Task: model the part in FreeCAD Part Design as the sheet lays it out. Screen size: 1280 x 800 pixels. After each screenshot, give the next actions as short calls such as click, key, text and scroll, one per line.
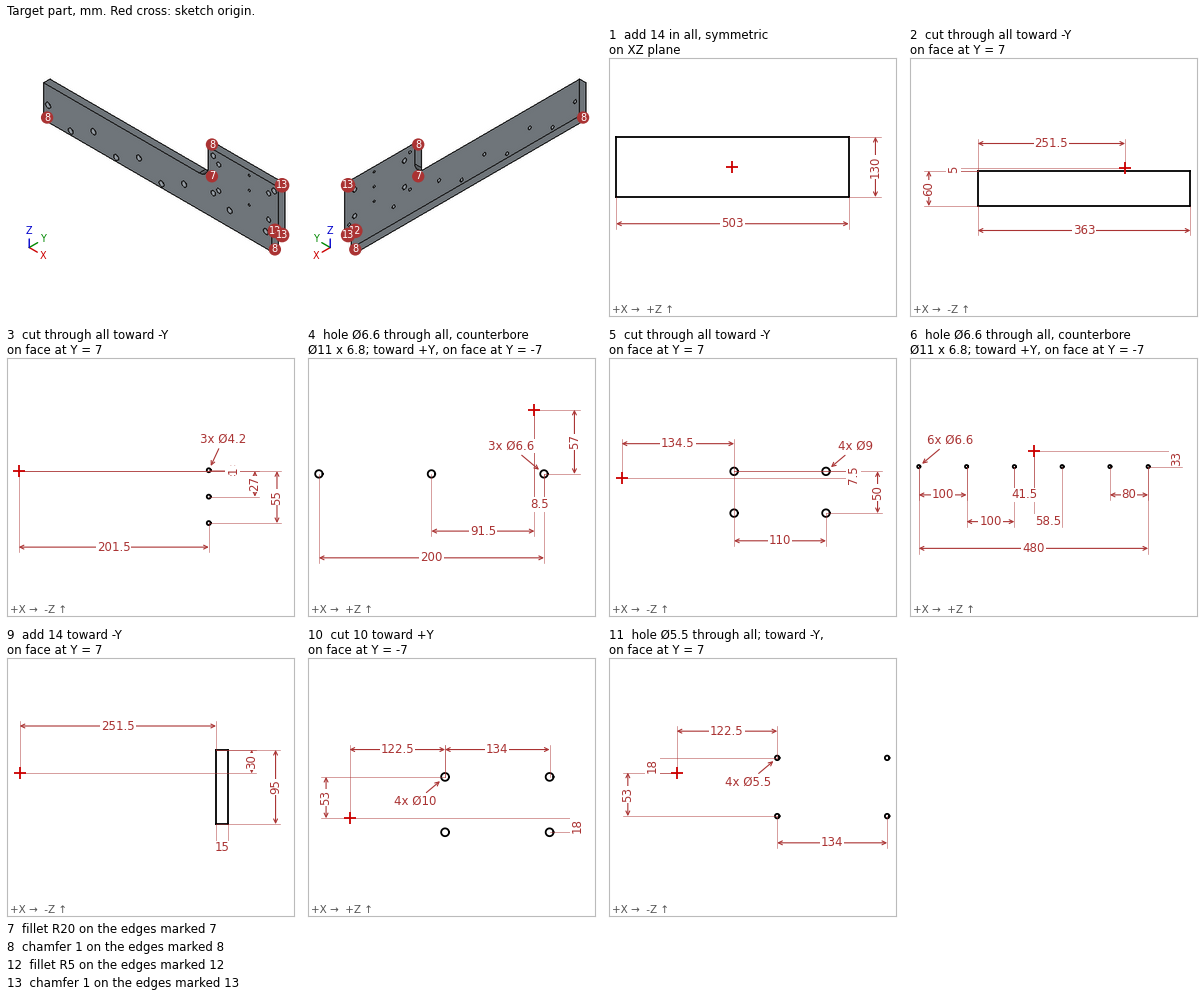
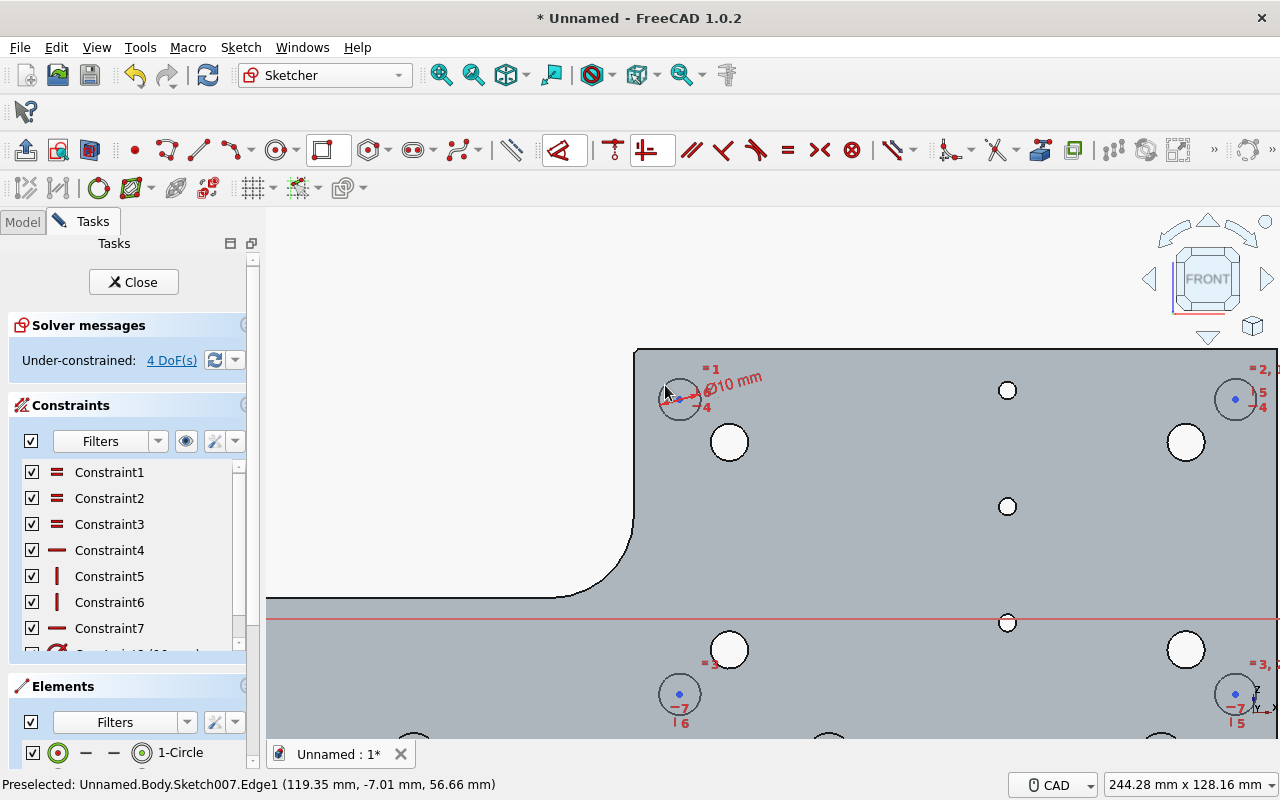
click(680, 400)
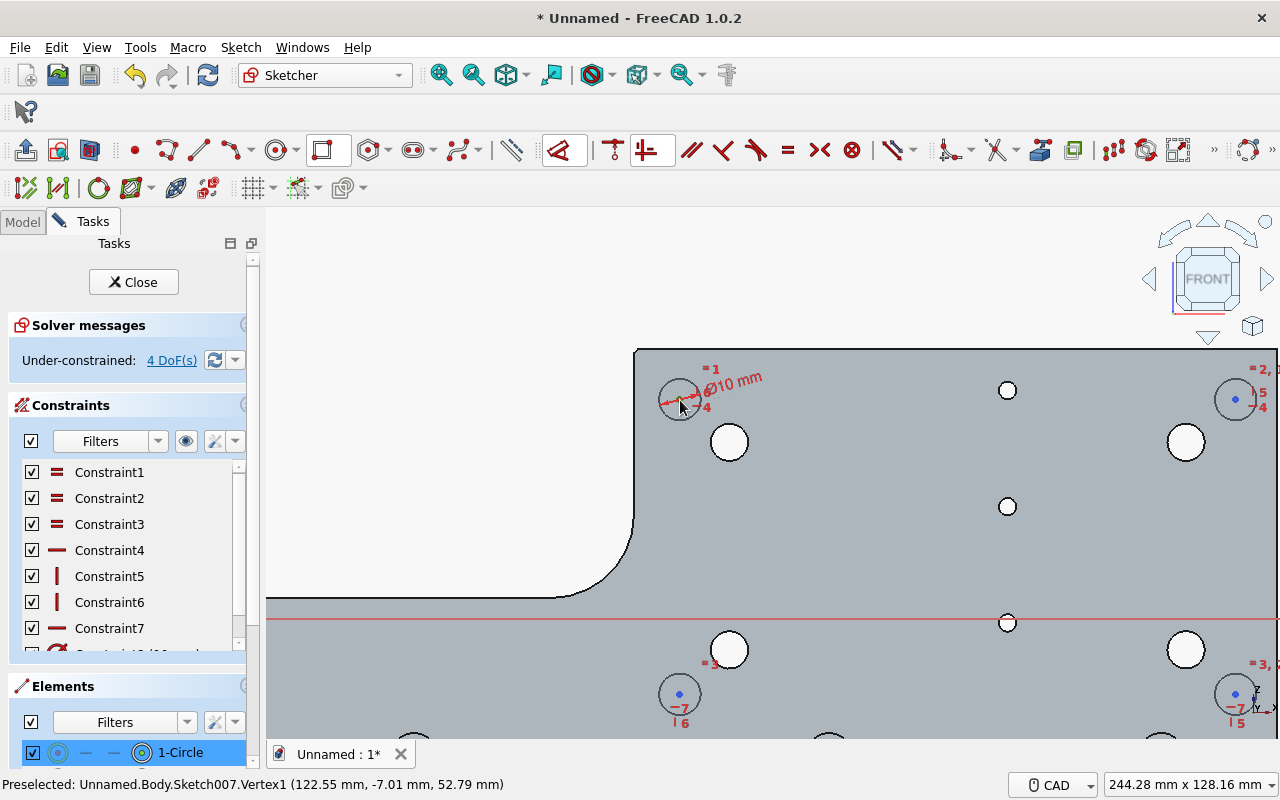
key(i)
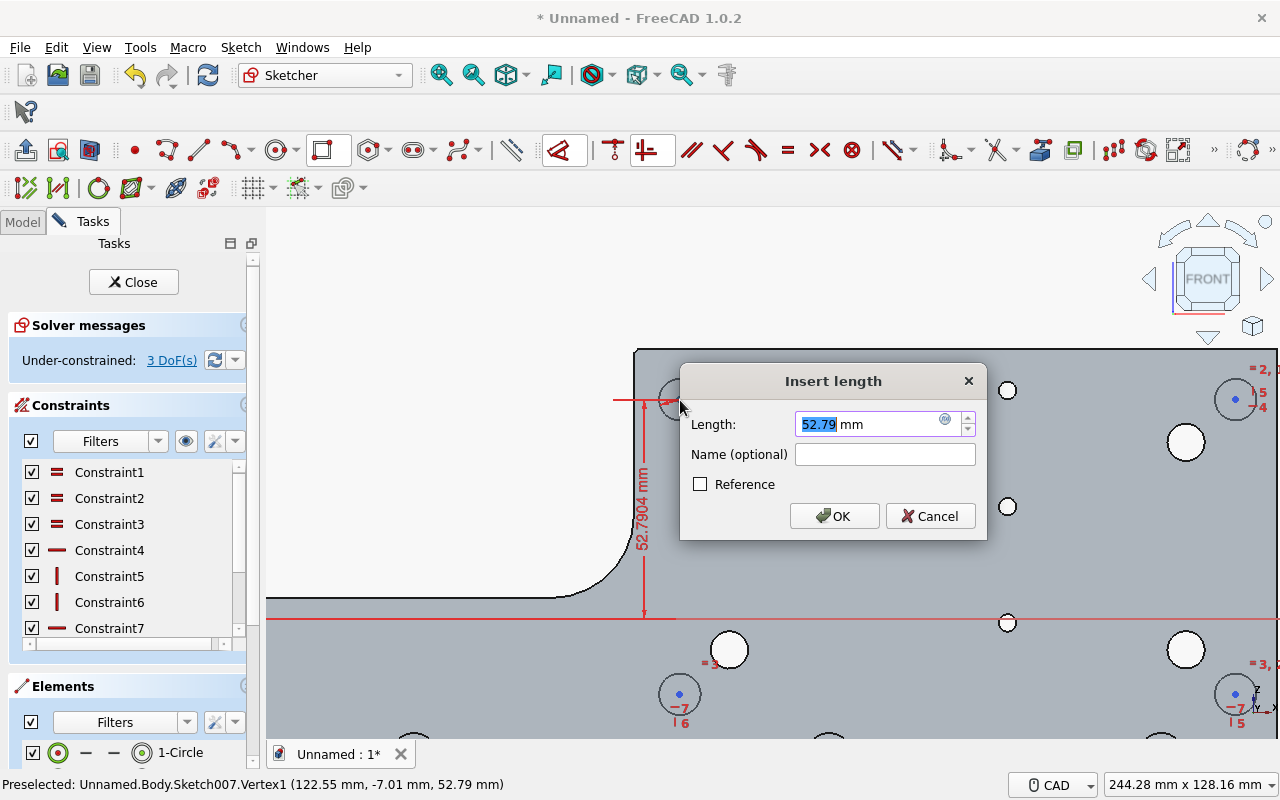
text(53)
key(Return)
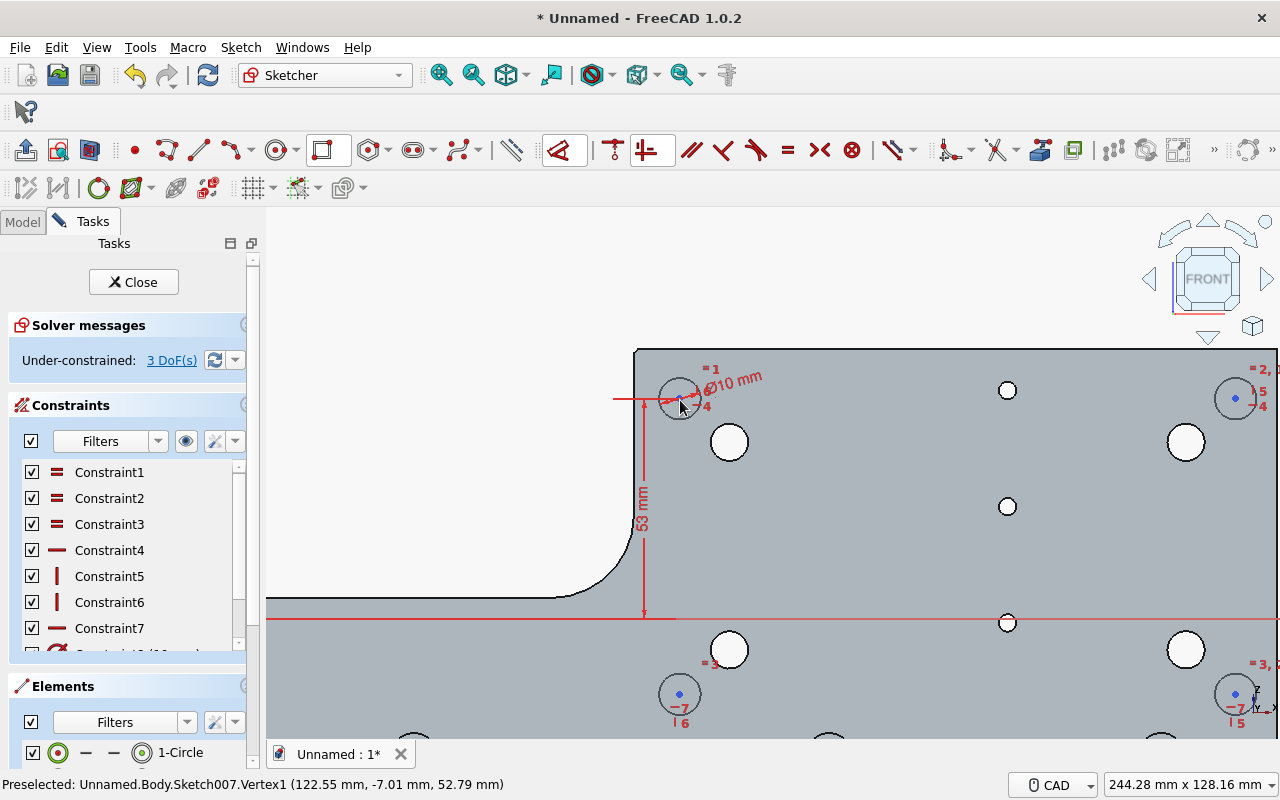
scroll(693, 384, down, 3)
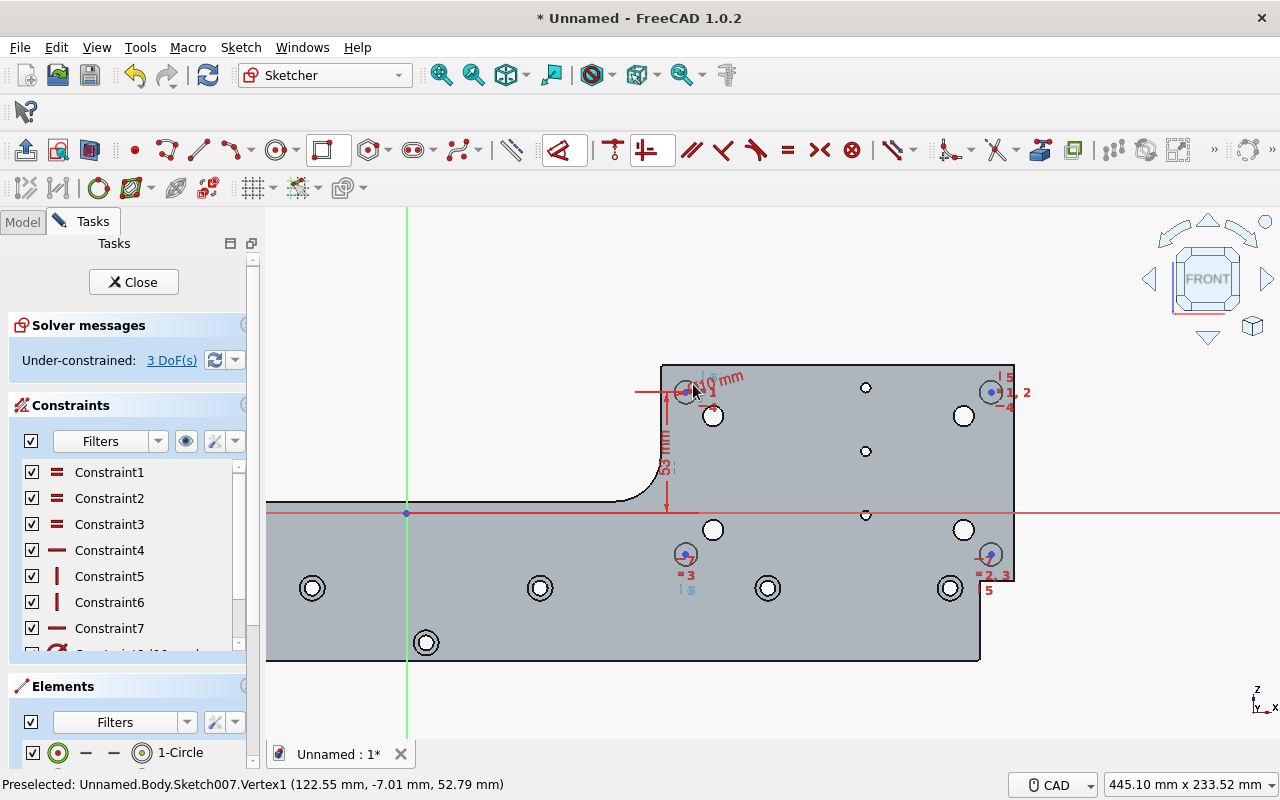
click(991, 554)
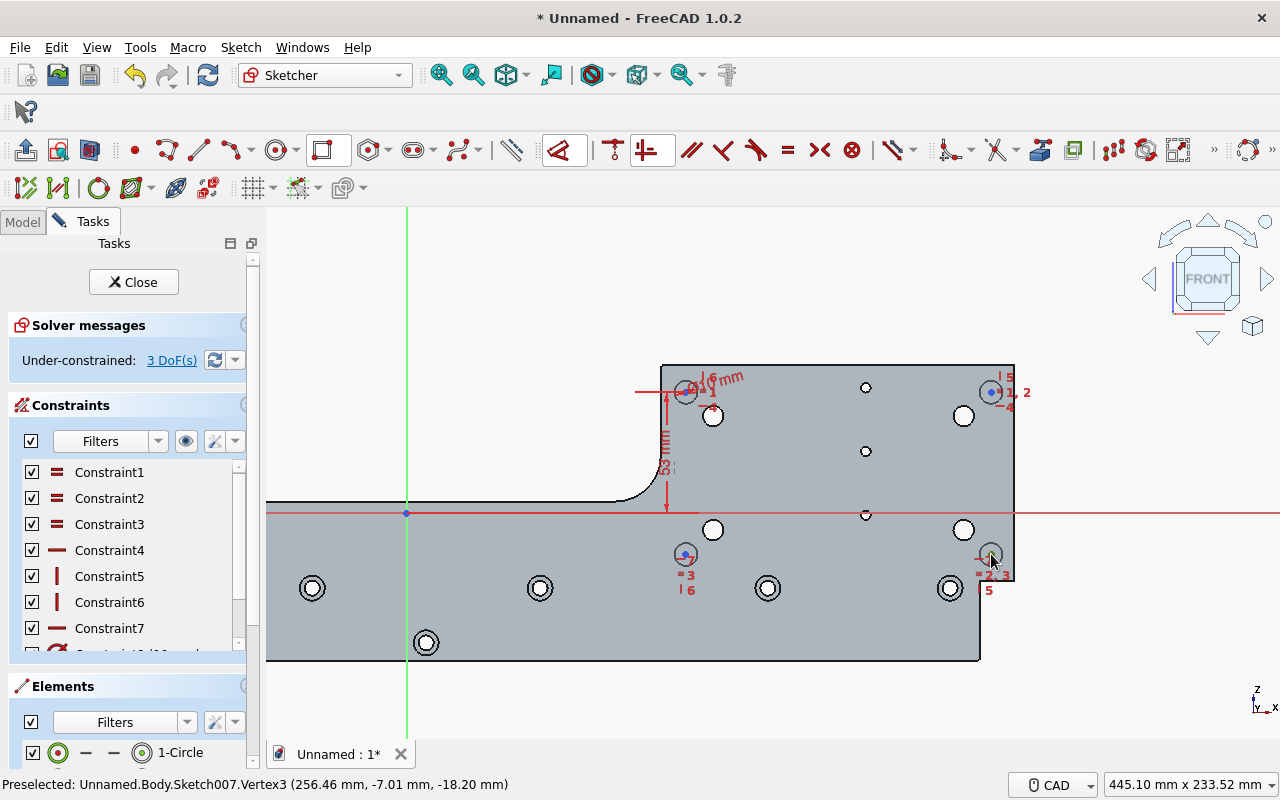
click(582, 150)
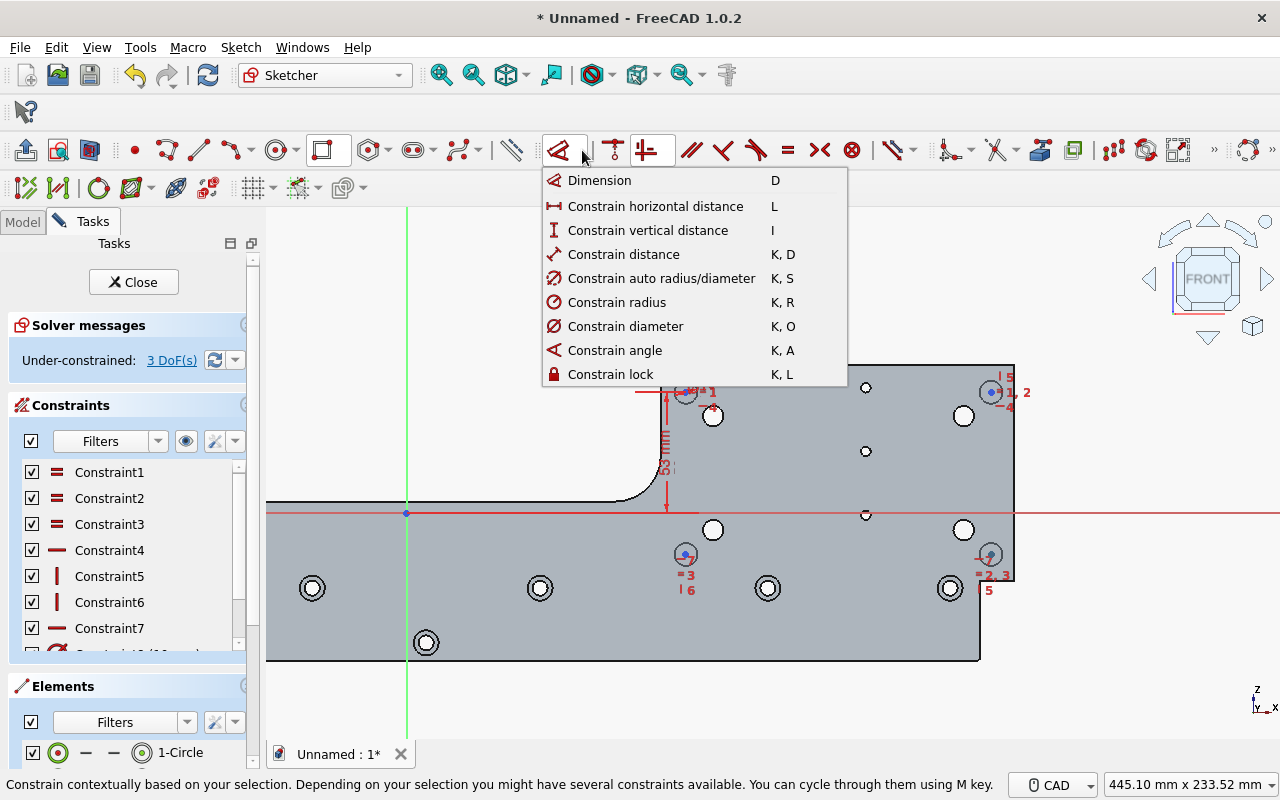
click(695, 230)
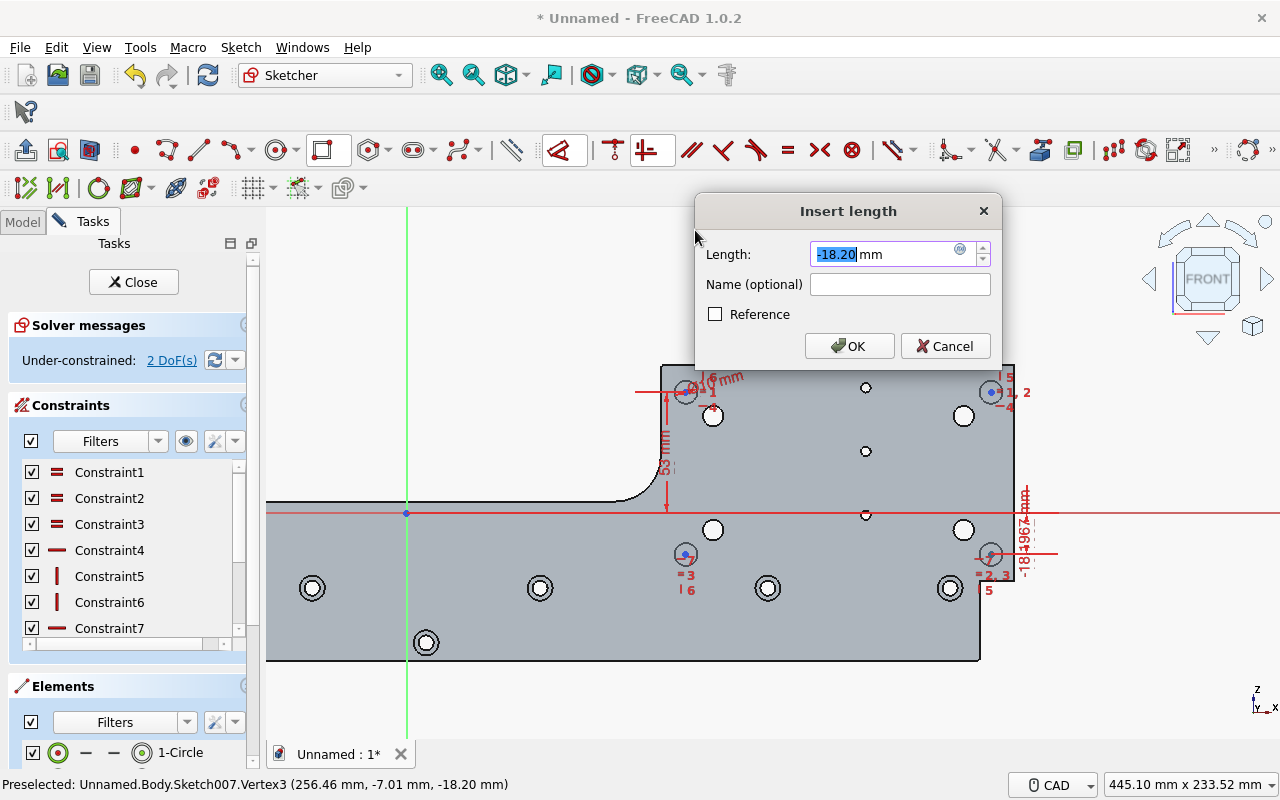
text(-18)
key(Return)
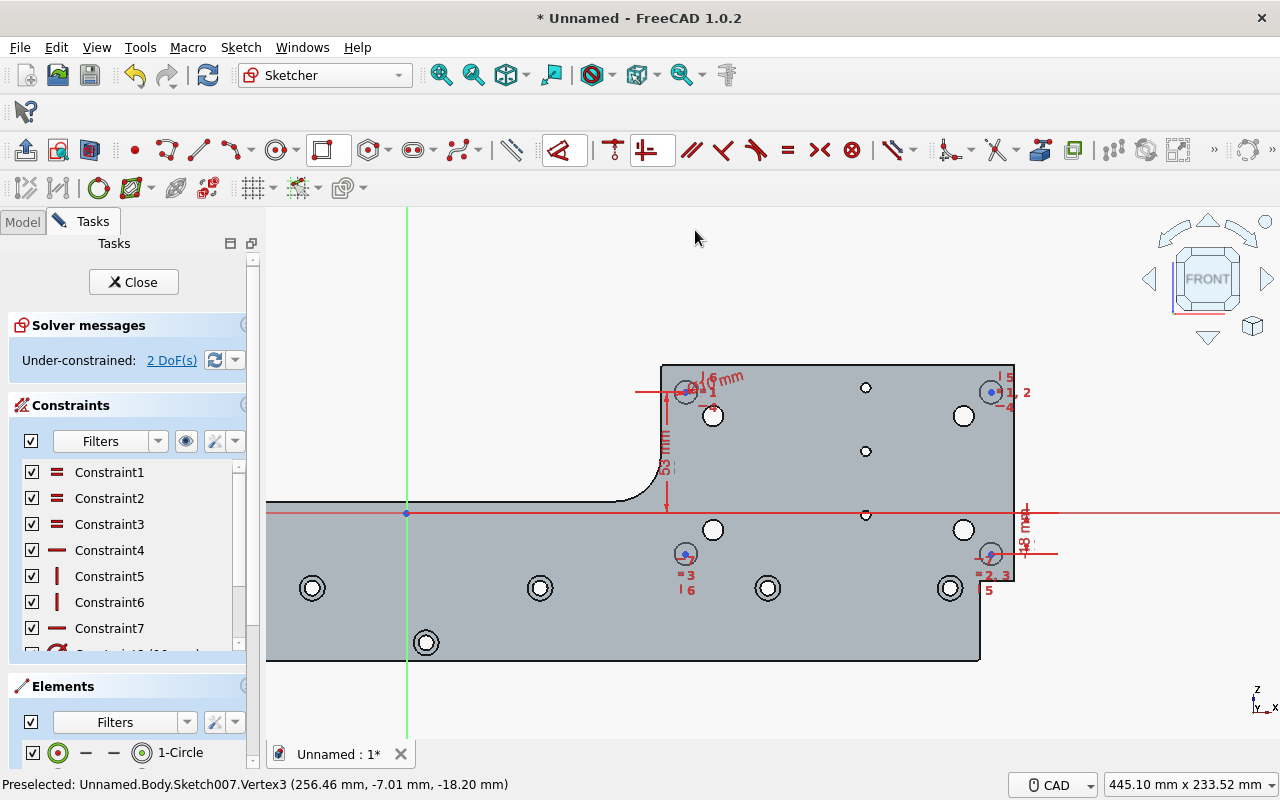
click(686, 392)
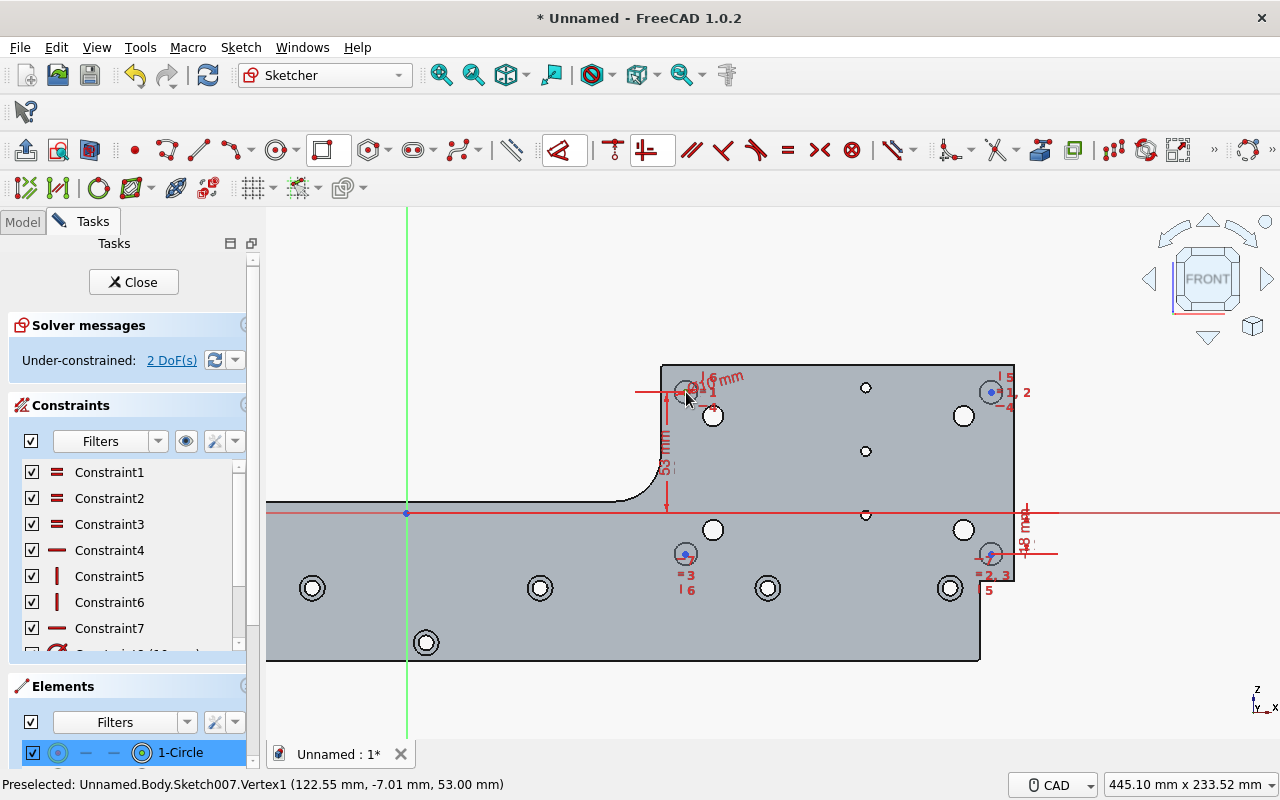
click(991, 392)